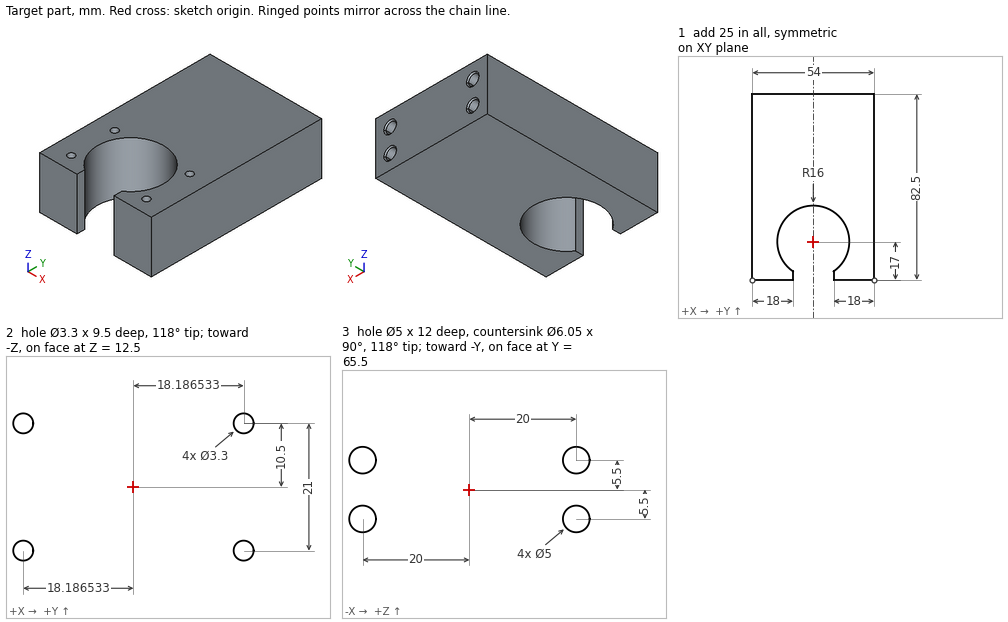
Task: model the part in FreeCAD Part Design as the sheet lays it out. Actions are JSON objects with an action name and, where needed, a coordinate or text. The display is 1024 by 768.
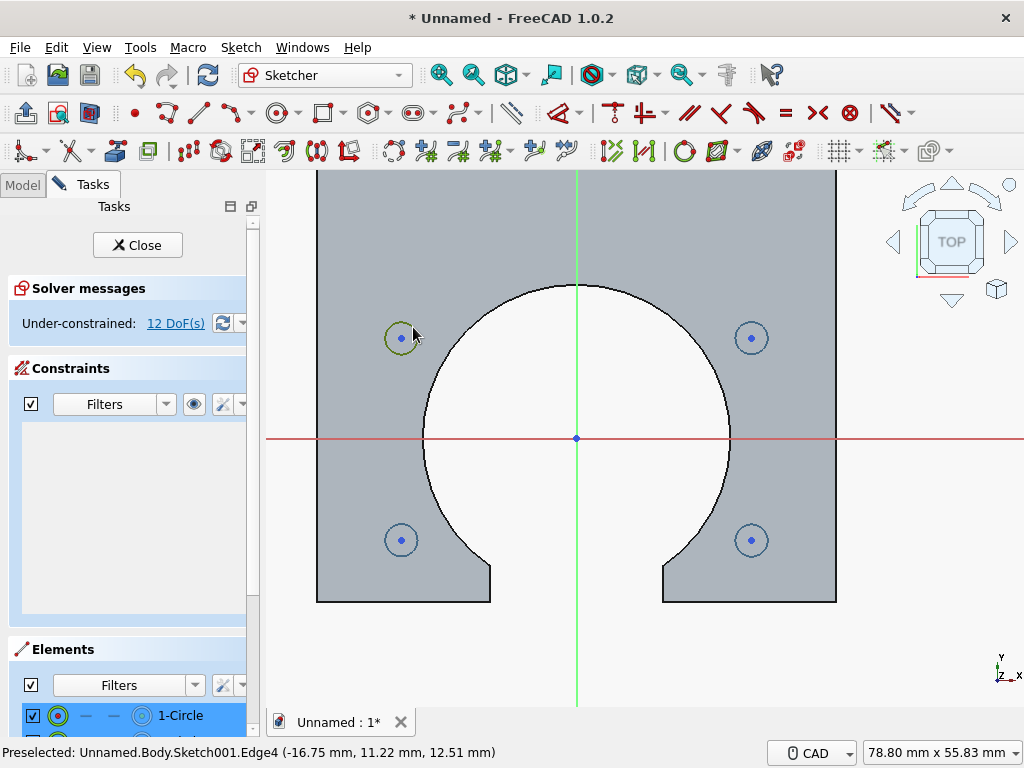
{"action": "left_click", "coordinate": [786, 114]}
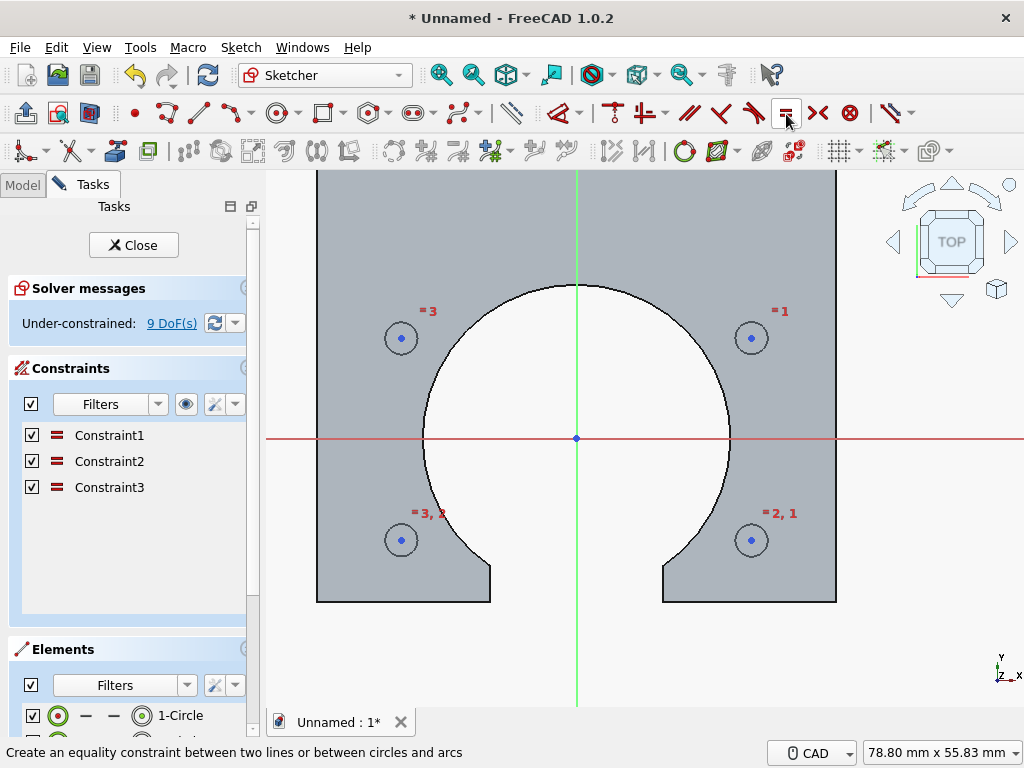
{"action": "left_click", "coordinate": [752, 338]}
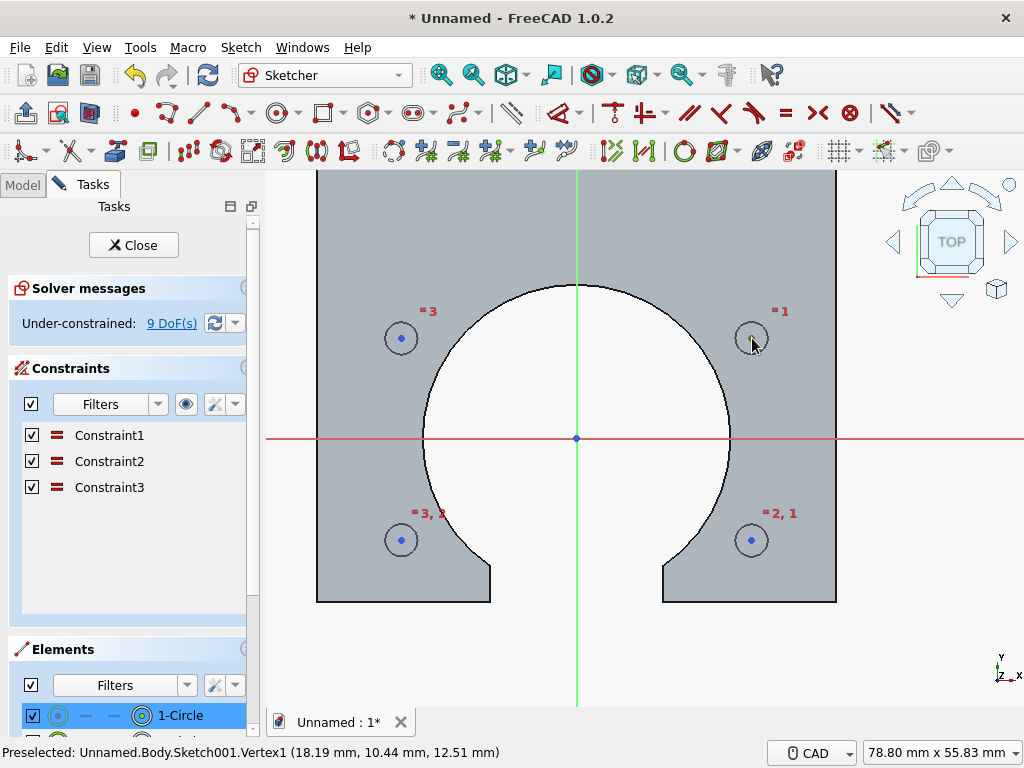
{"action": "left_click", "coordinate": [752, 541]}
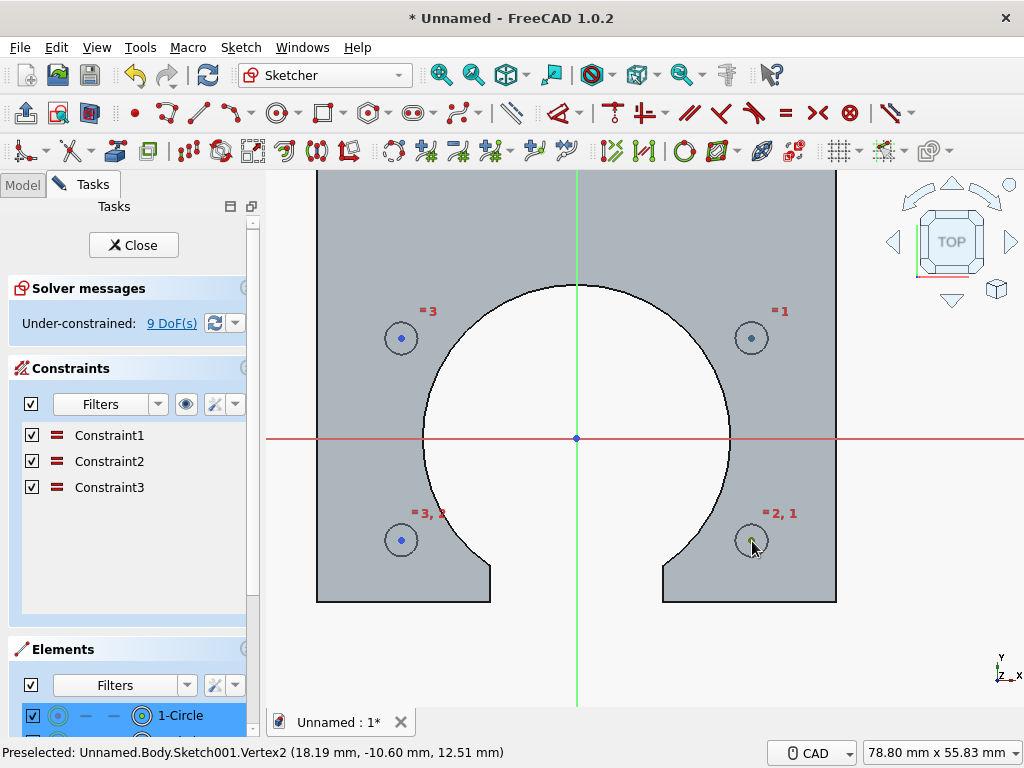
{"action": "key", "text": "v"}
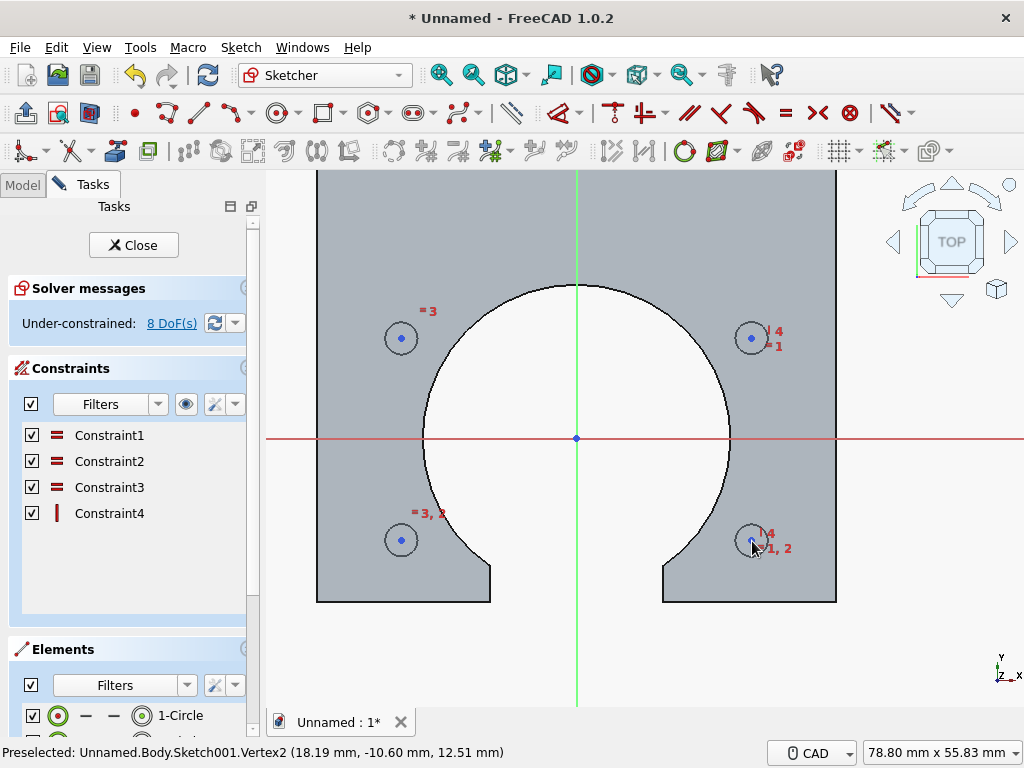
{"action": "left_click", "coordinate": [752, 541]}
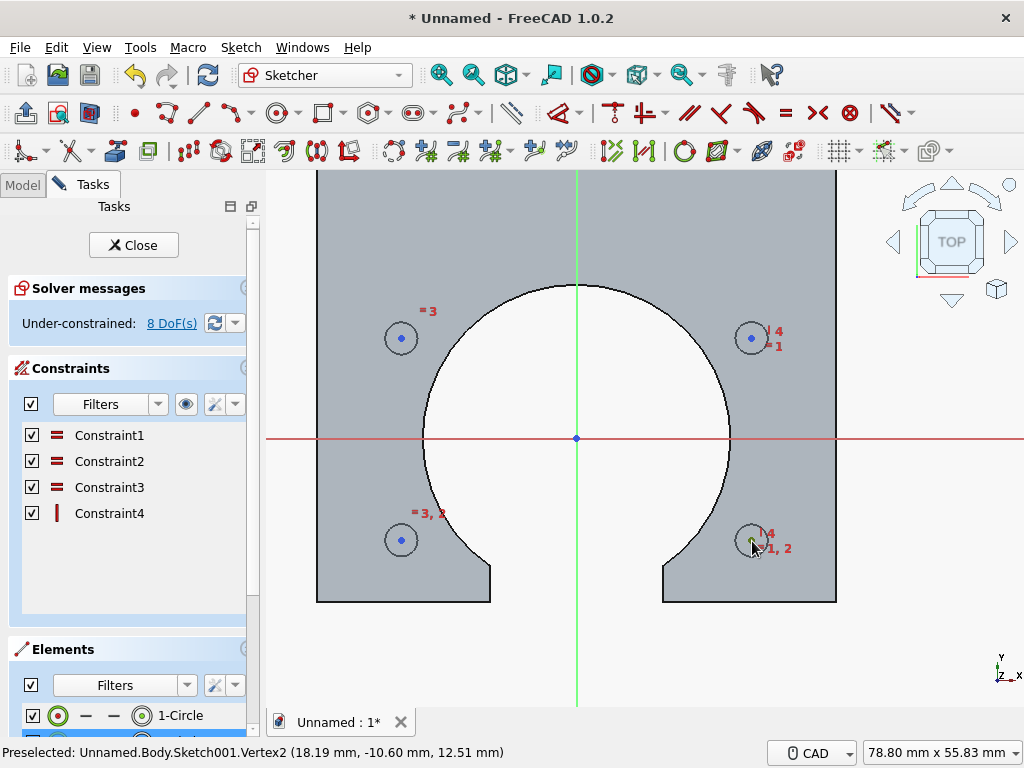
{"action": "left_click", "coordinate": [401, 540]}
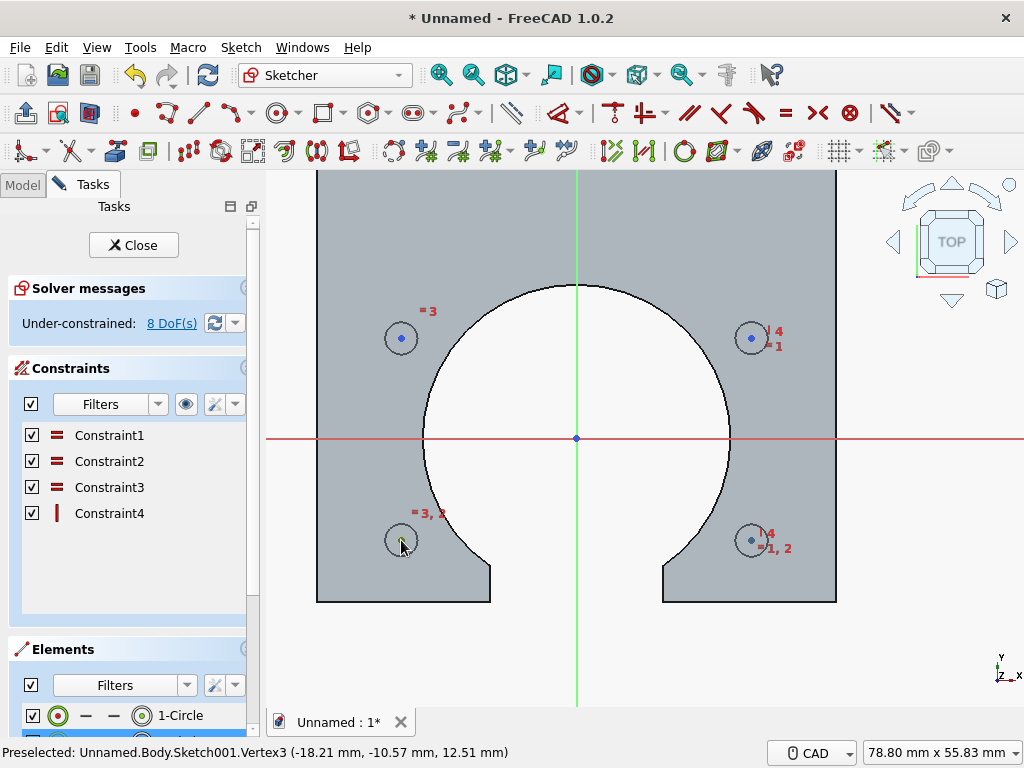
{"action": "left_click", "coordinate": [668, 114]}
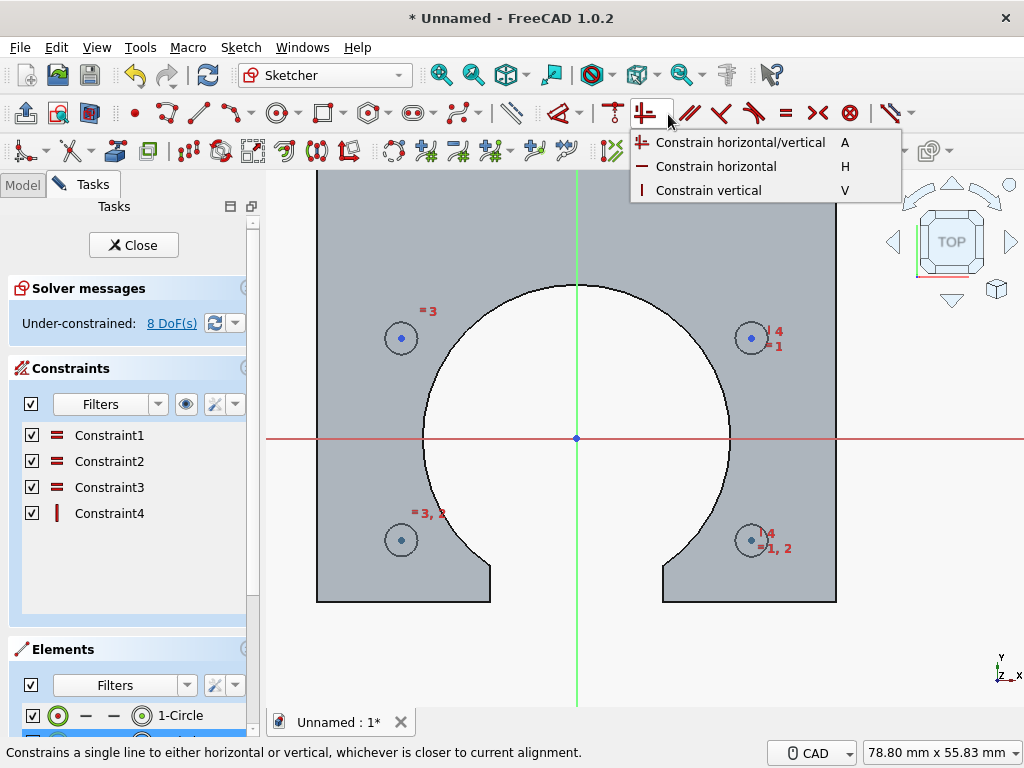
{"action": "left_click", "coordinate": [766, 166]}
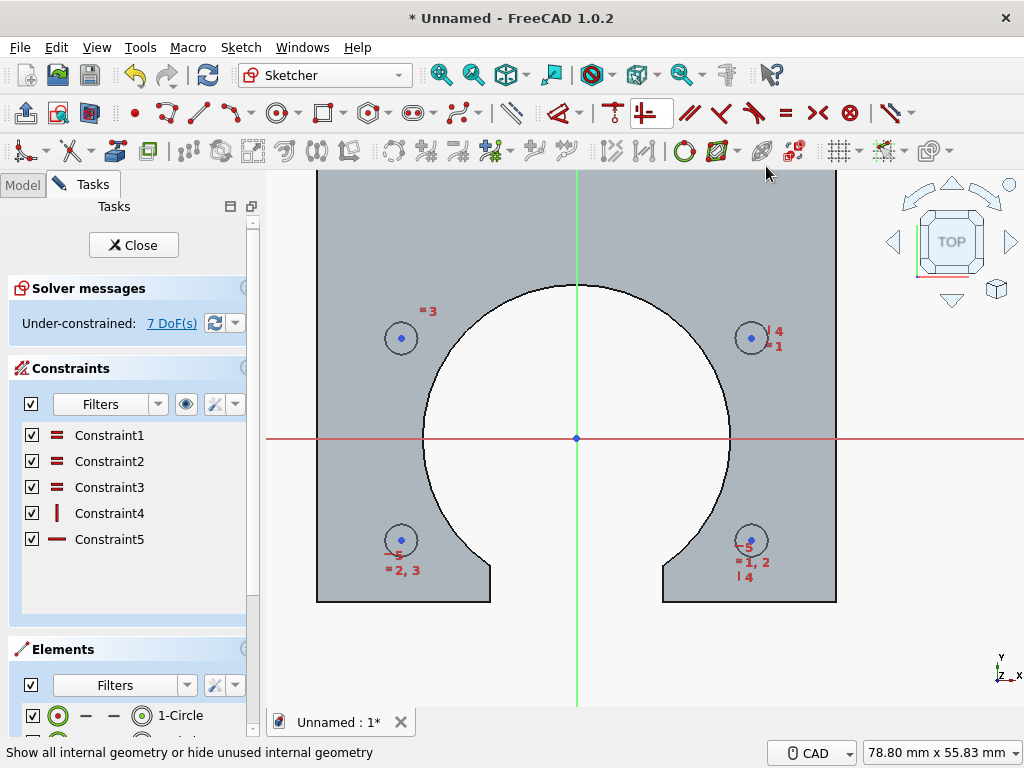
{"action": "left_click", "coordinate": [401, 541]}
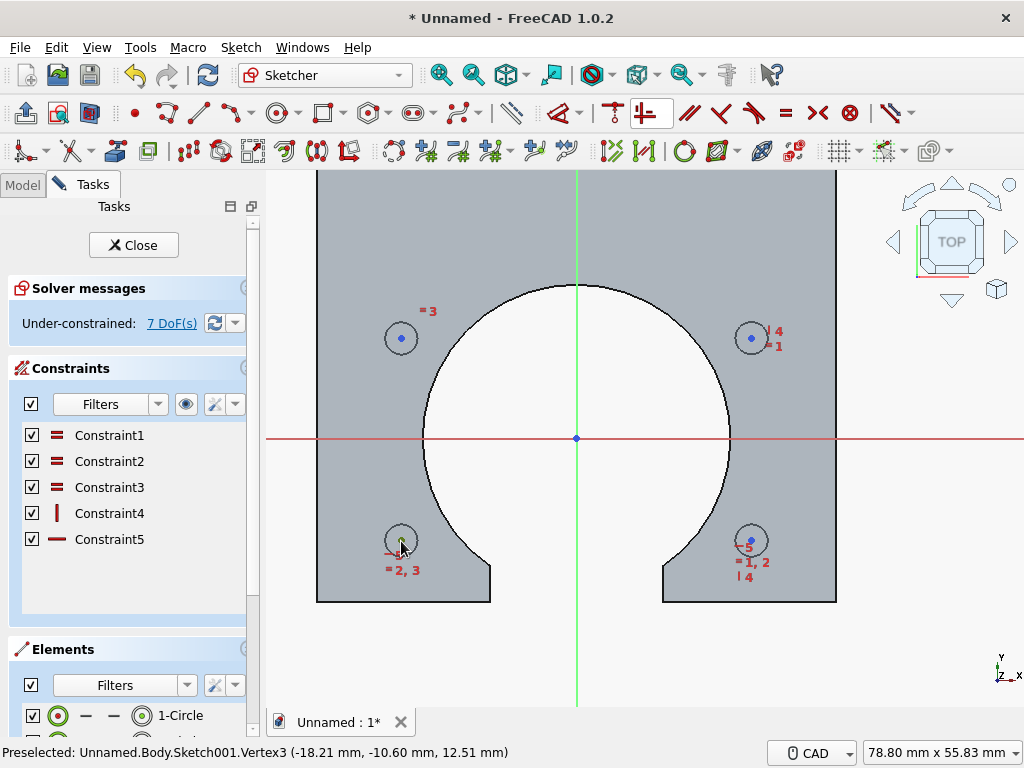
{"action": "left_click", "coordinate": [401, 338]}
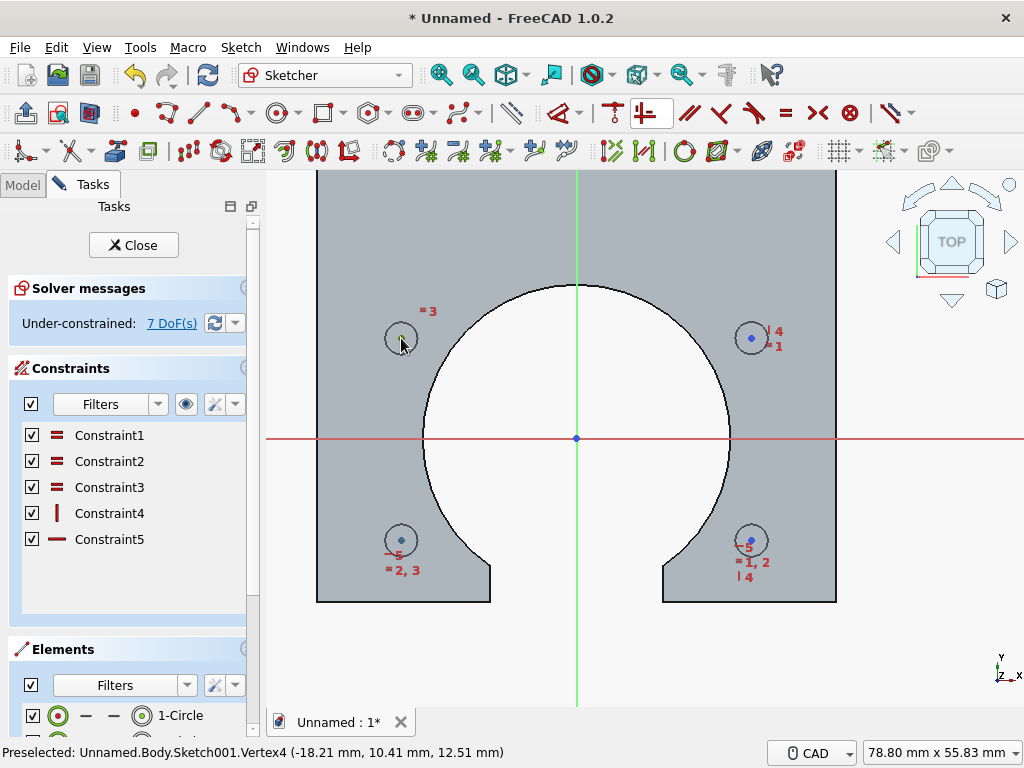
{"action": "key", "text": "v"}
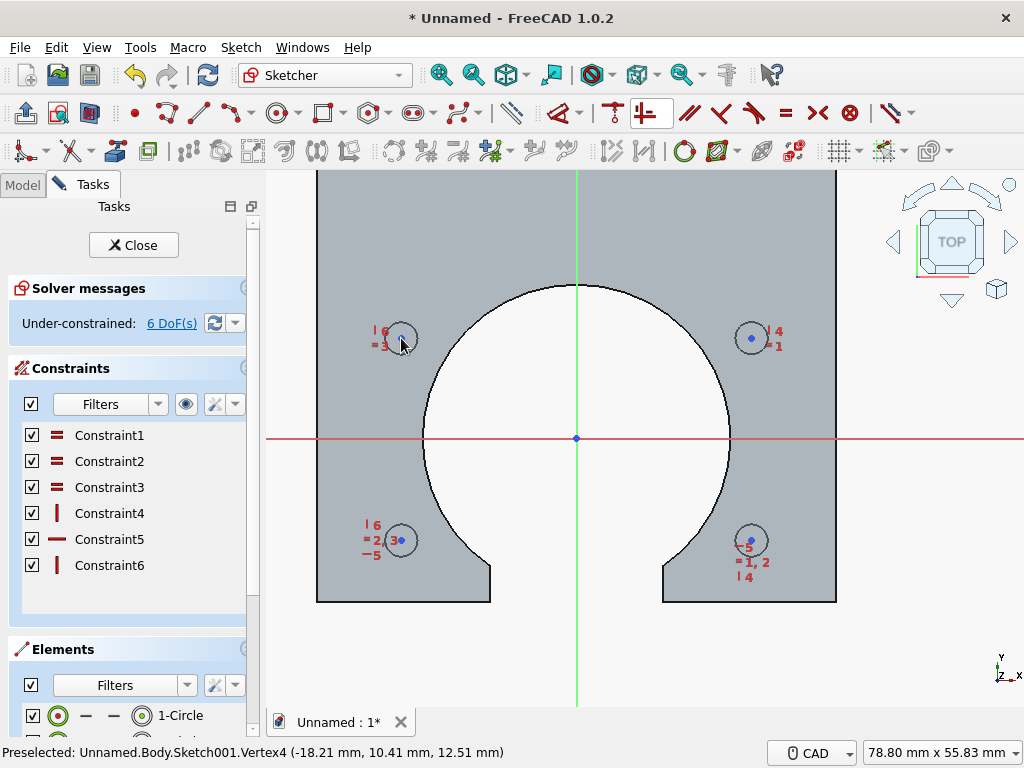
{"action": "left_click", "coordinate": [752, 338]}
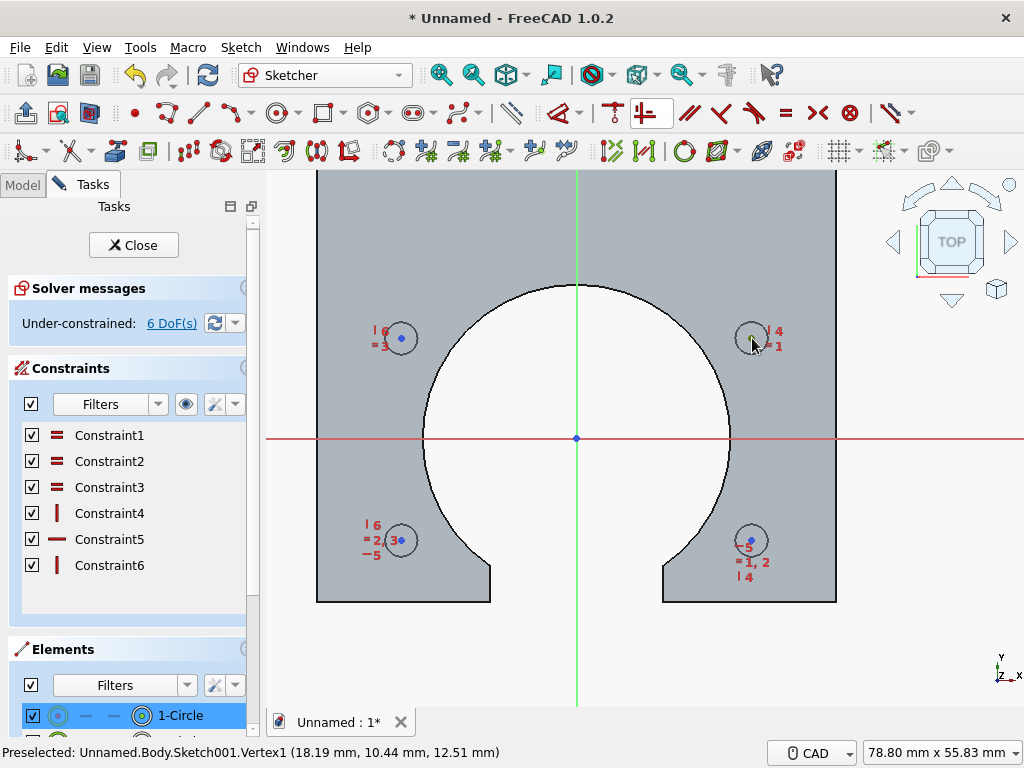
{"action": "left_click", "coordinate": [401, 338]}